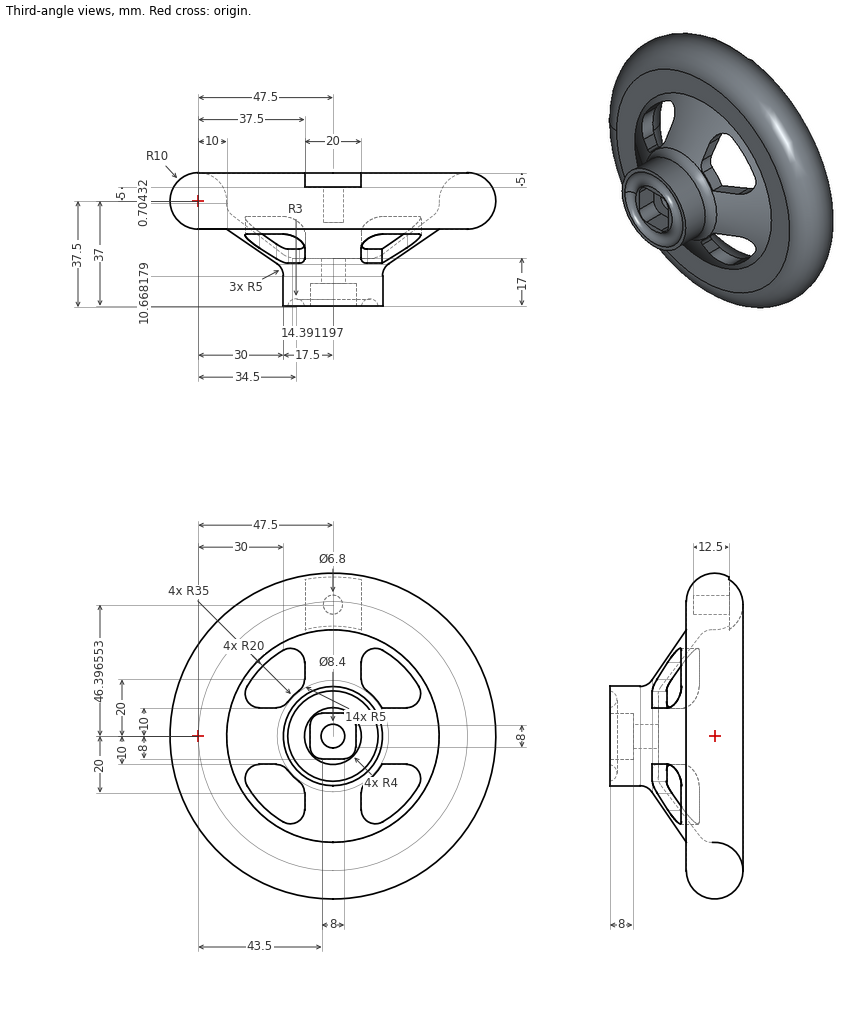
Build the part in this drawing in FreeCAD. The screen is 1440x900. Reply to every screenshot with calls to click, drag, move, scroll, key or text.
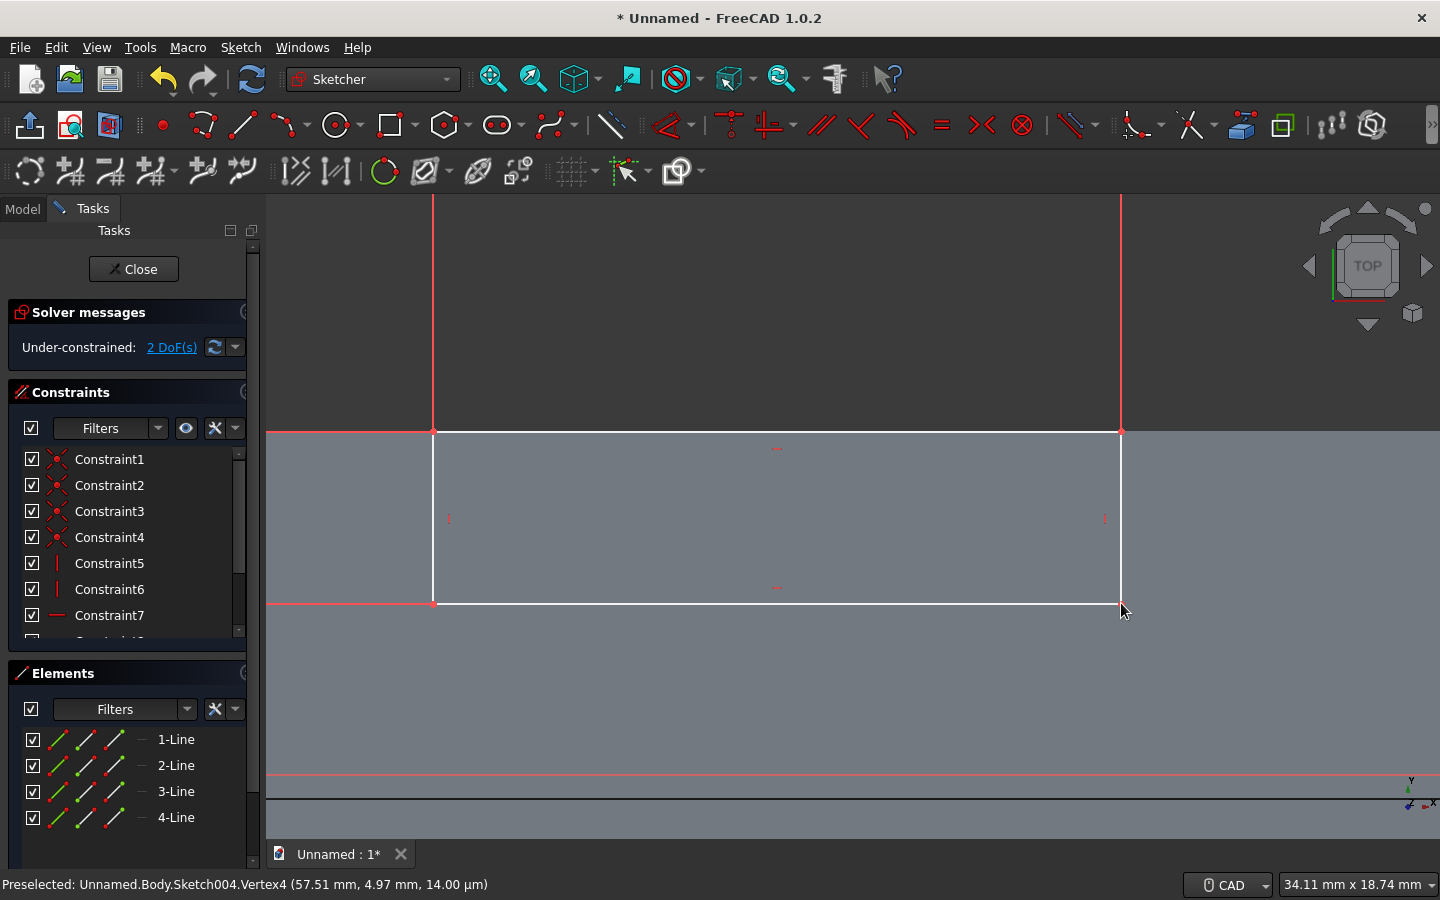
click(666, 126)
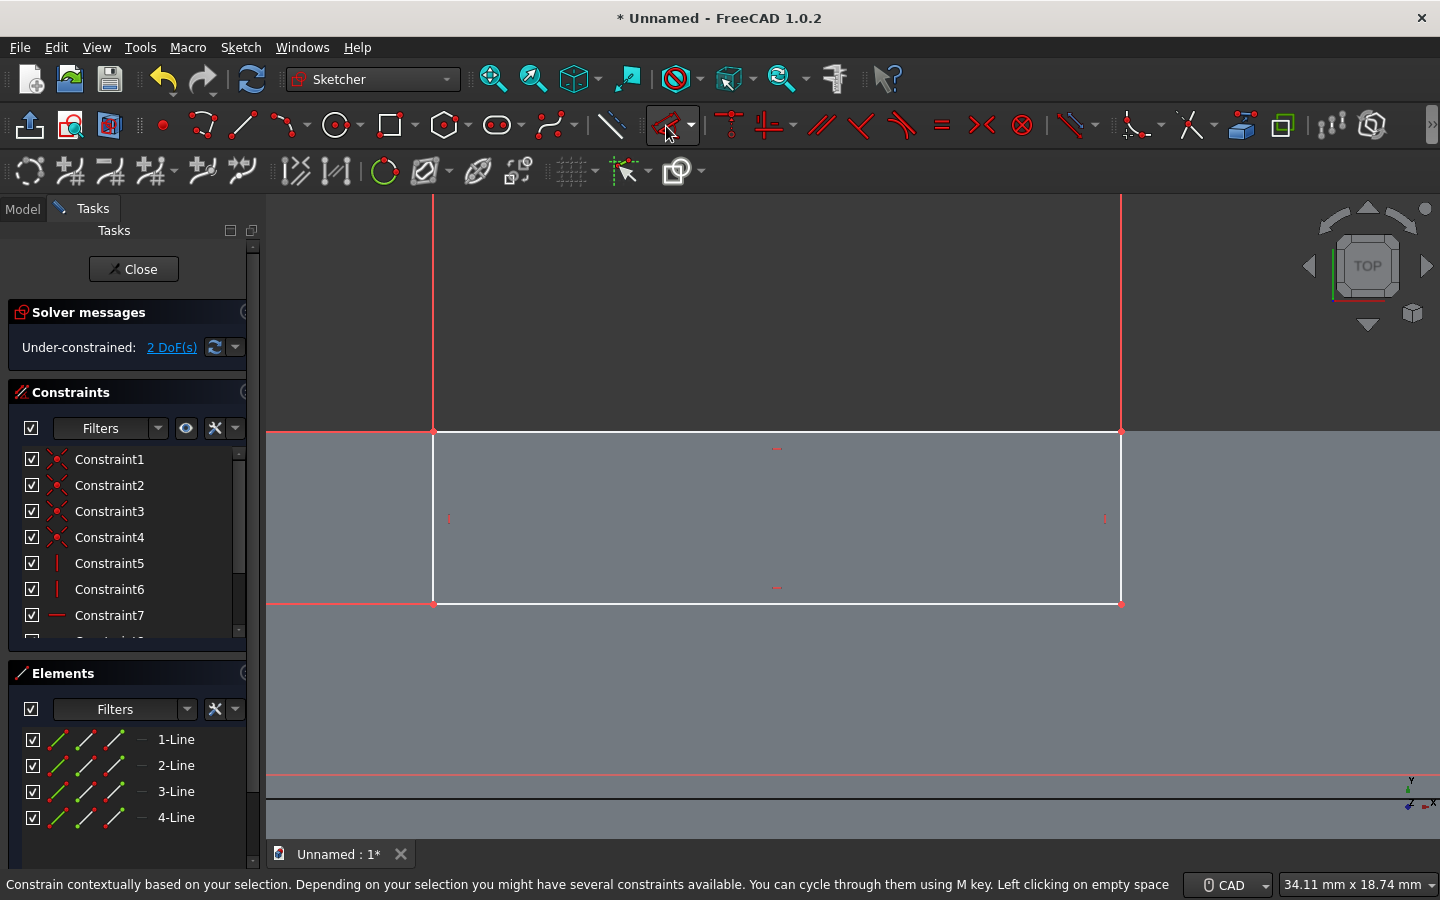
click(433, 604)
click(467, 690)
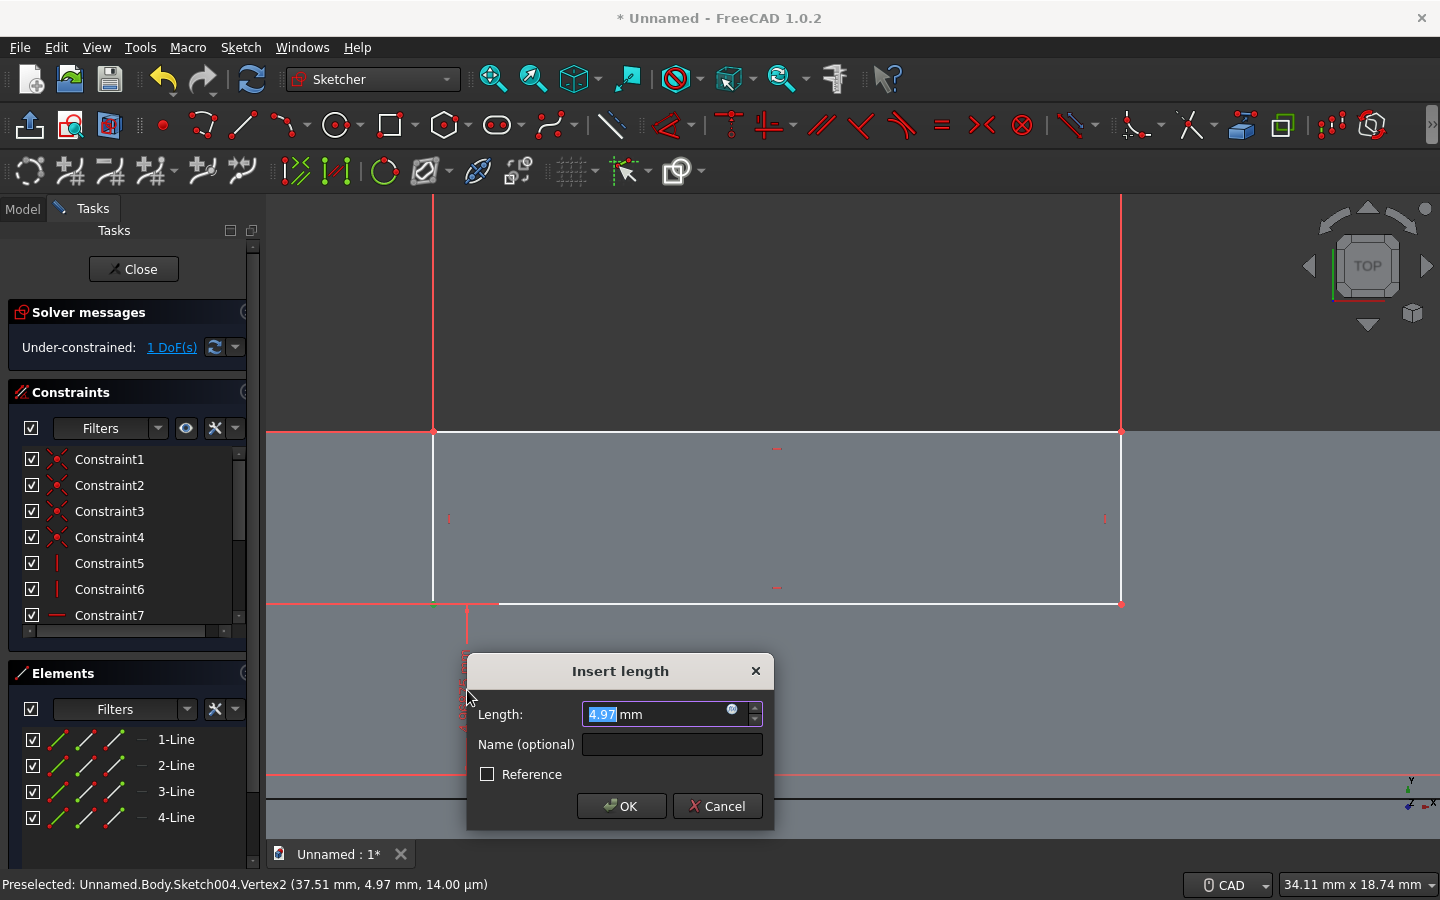
text(5)
key(Return)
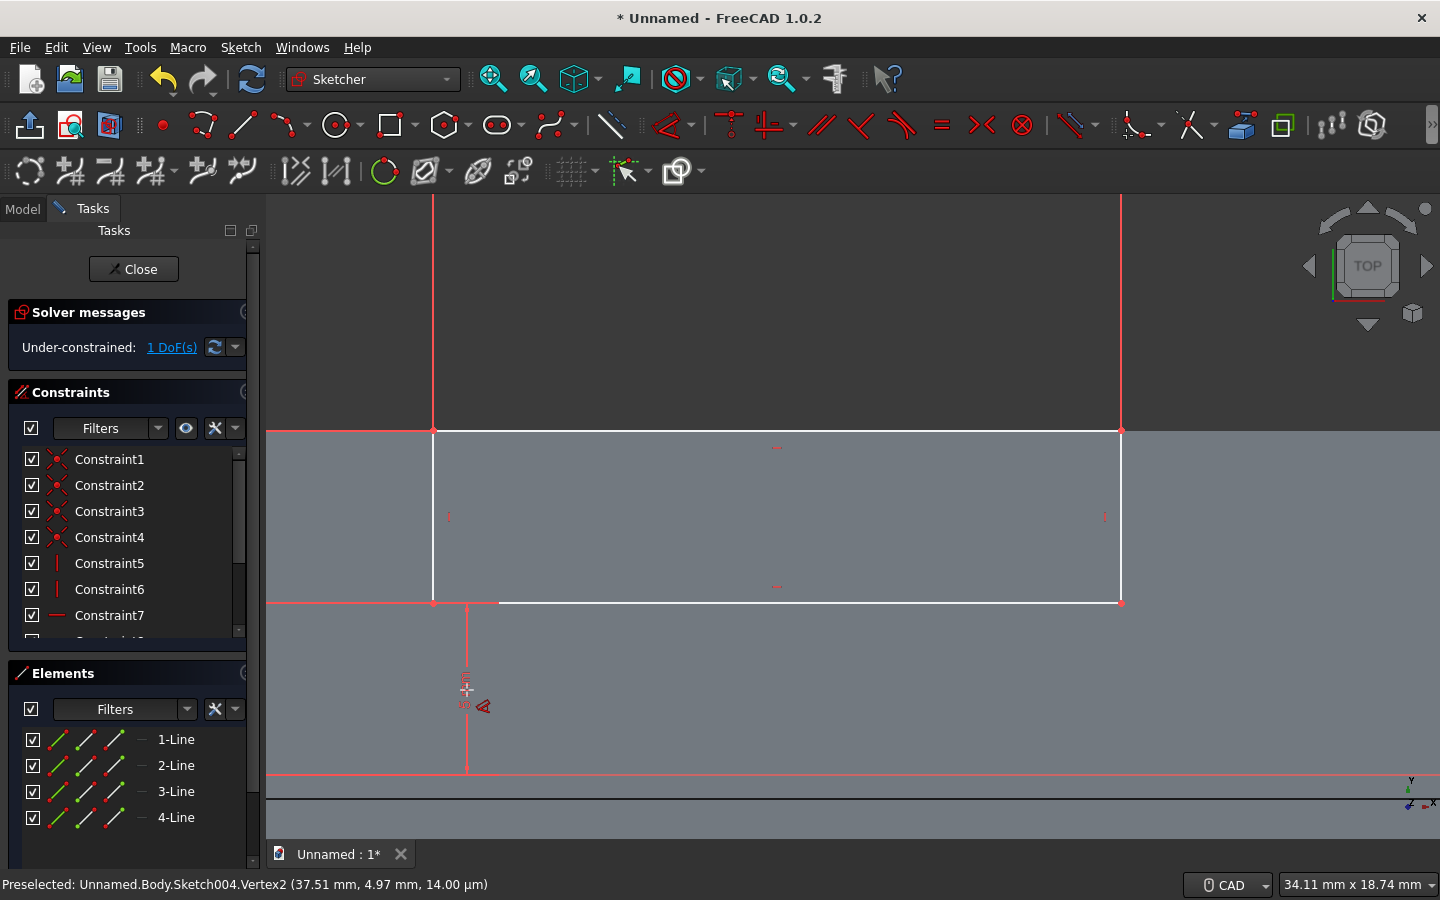
click(433, 431)
click(364, 809)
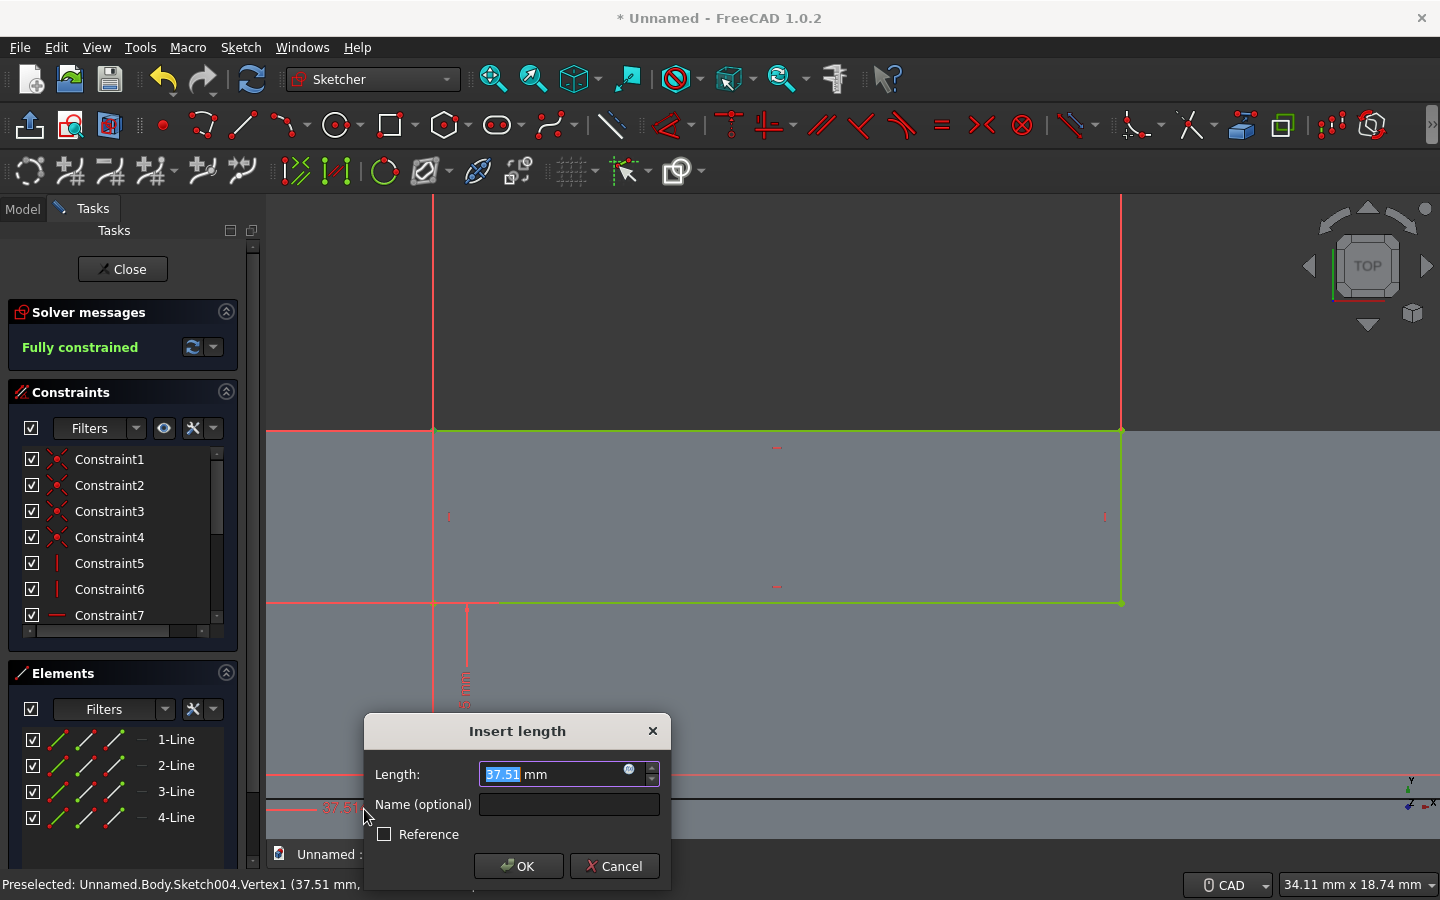
text(37.5)
key(Return)
key(Escape)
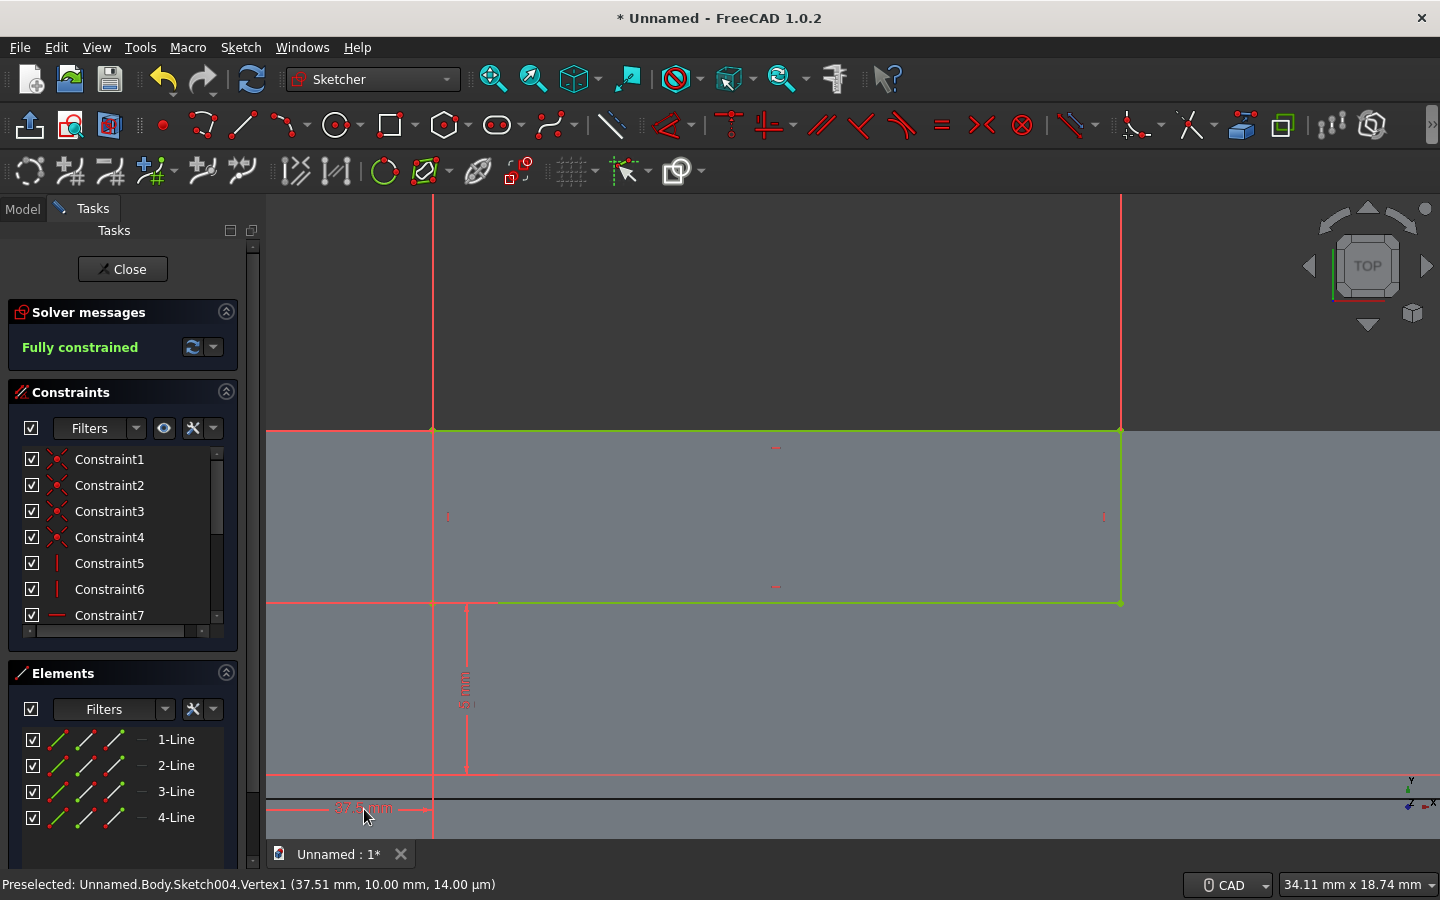
click(123, 269)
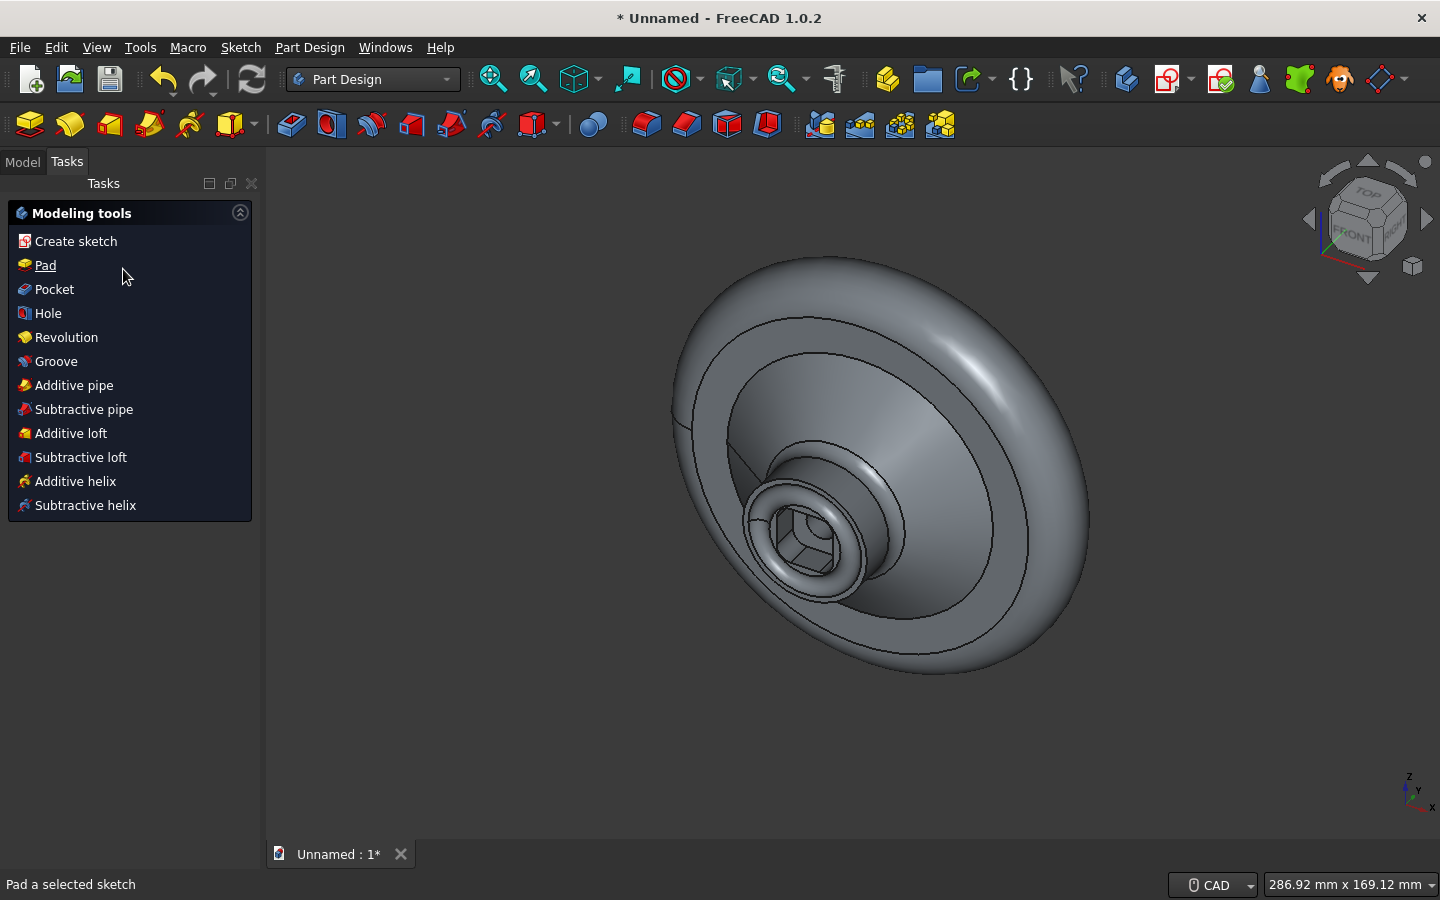
click(292, 124)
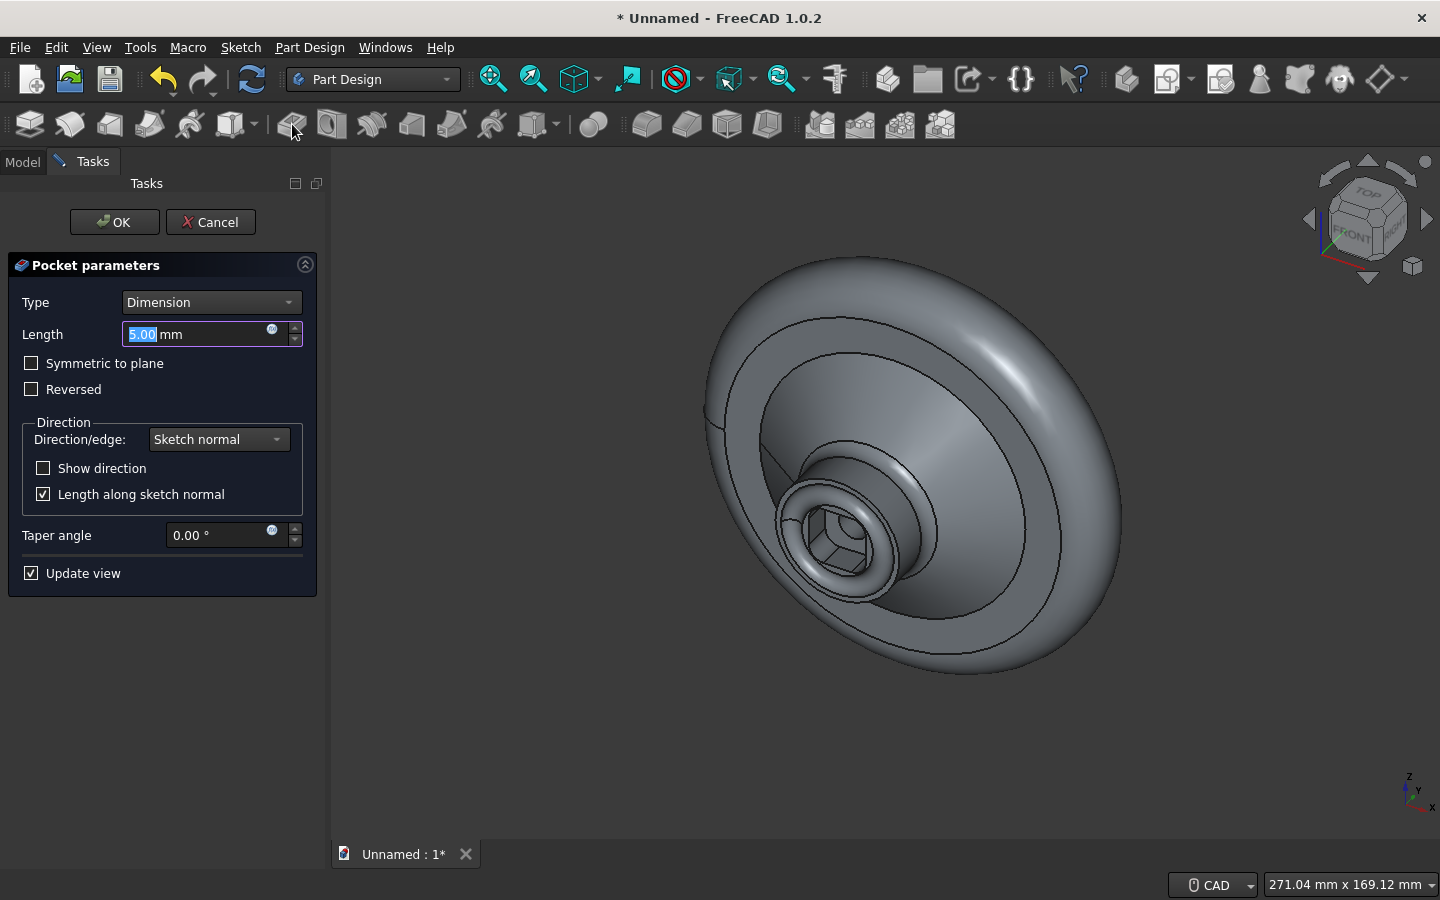
click(212, 302)